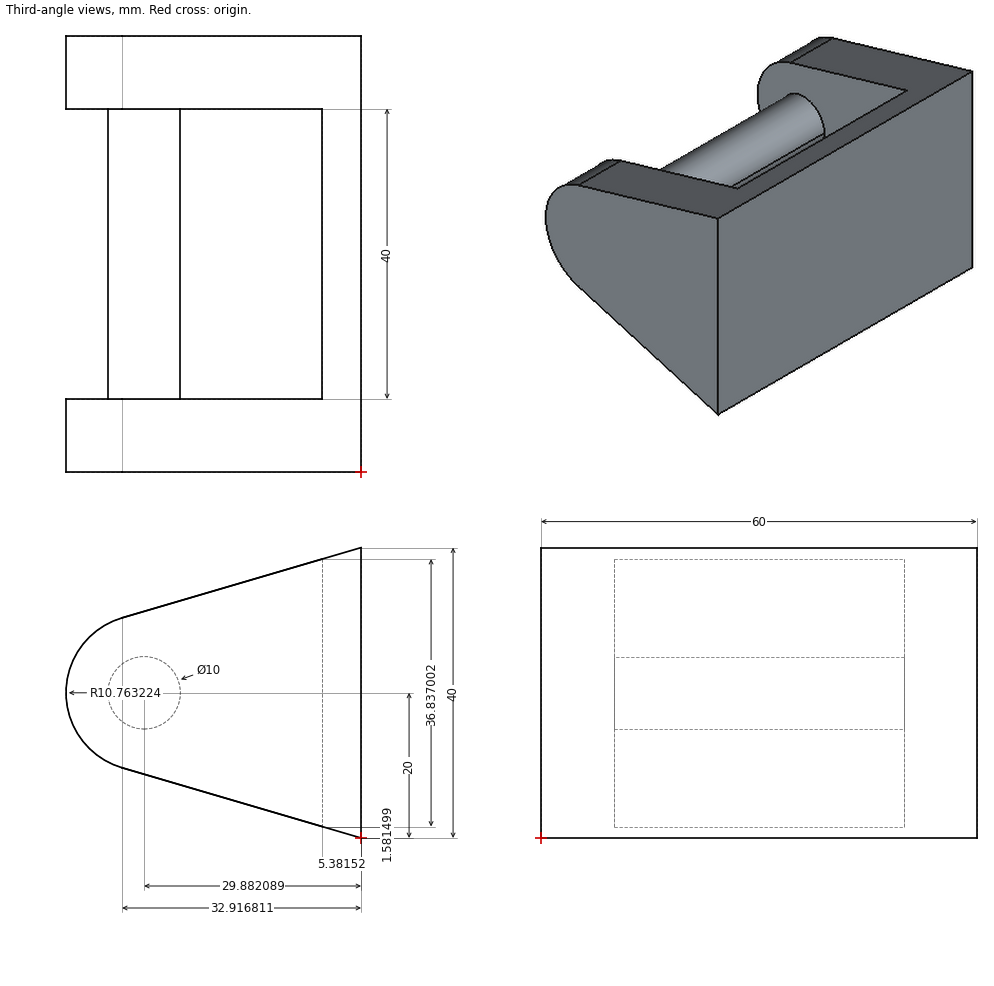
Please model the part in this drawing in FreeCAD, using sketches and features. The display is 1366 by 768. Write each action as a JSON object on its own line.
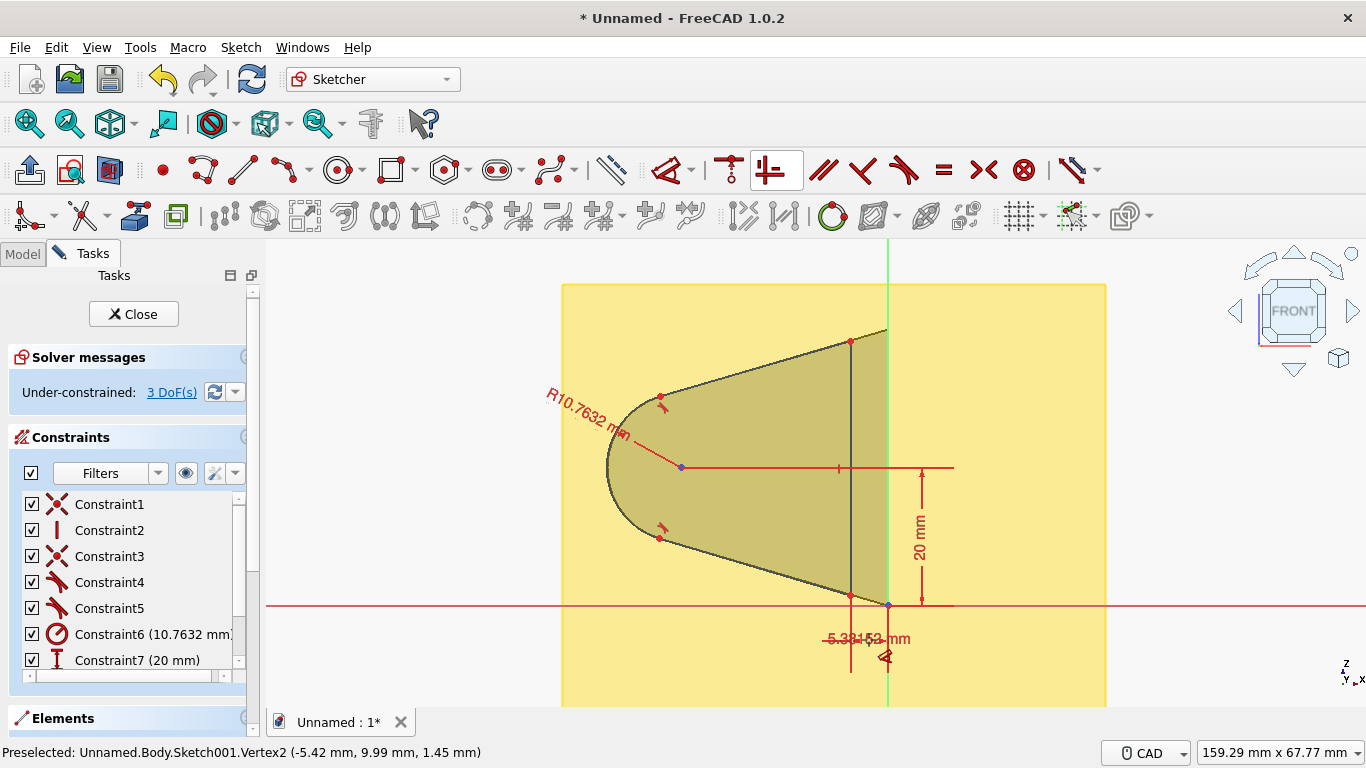
{"action": "left_click", "coordinate": [851, 519]}
{"action": "left_click", "coordinate": [817, 468]}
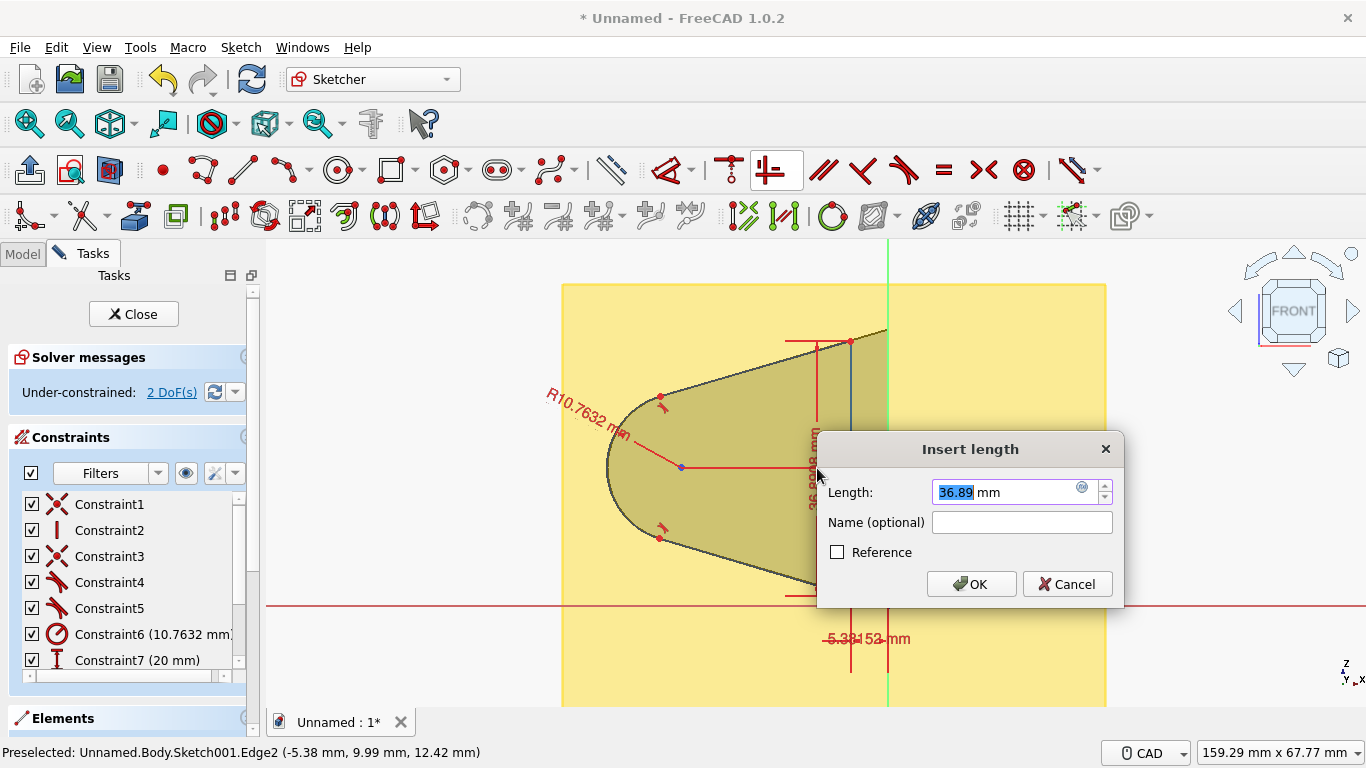
{"action": "type", "text": "36.837002"}
{"action": "key", "text": "Return"}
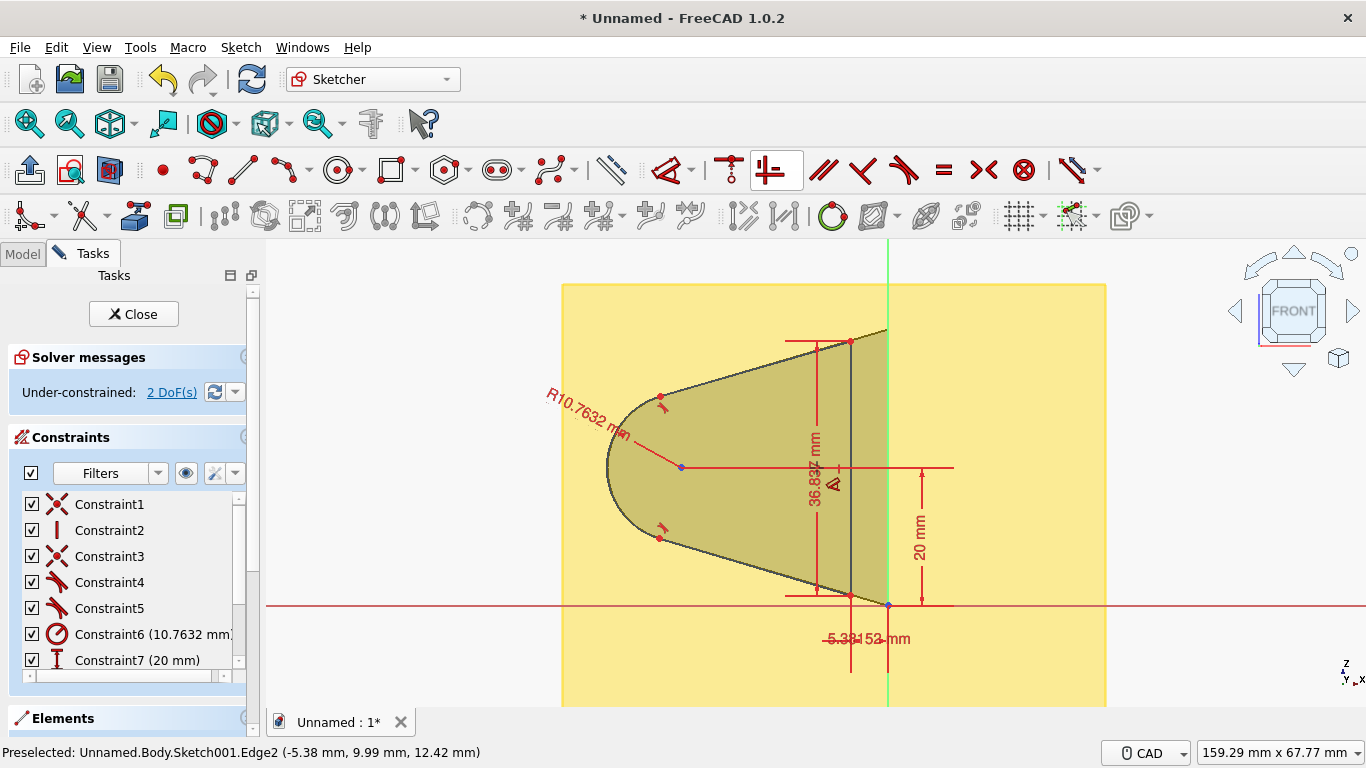
{"action": "scroll", "coordinate": [851, 596], "scroll_direction": "up", "scroll_amount": 7}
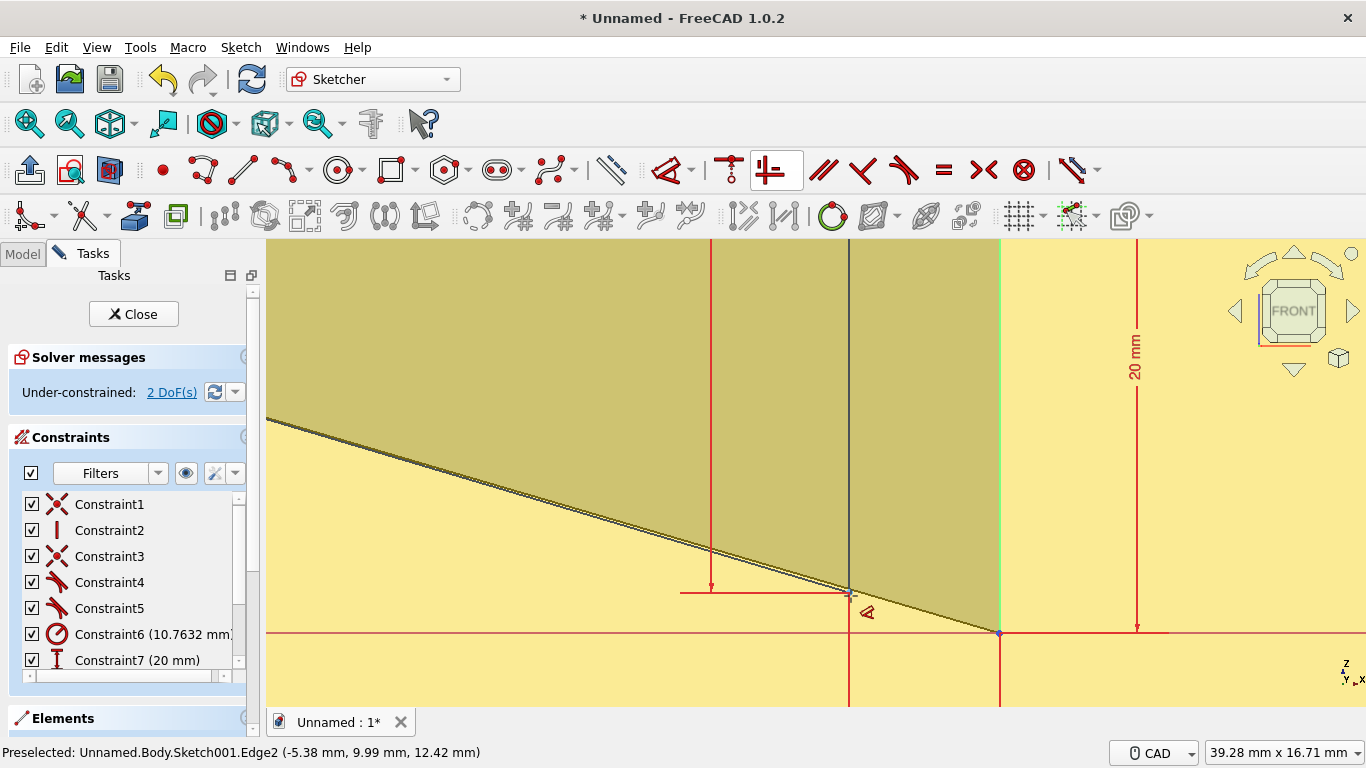
{"action": "left_click", "coordinate": [849, 593]}
{"action": "left_click", "coordinate": [1034, 613]}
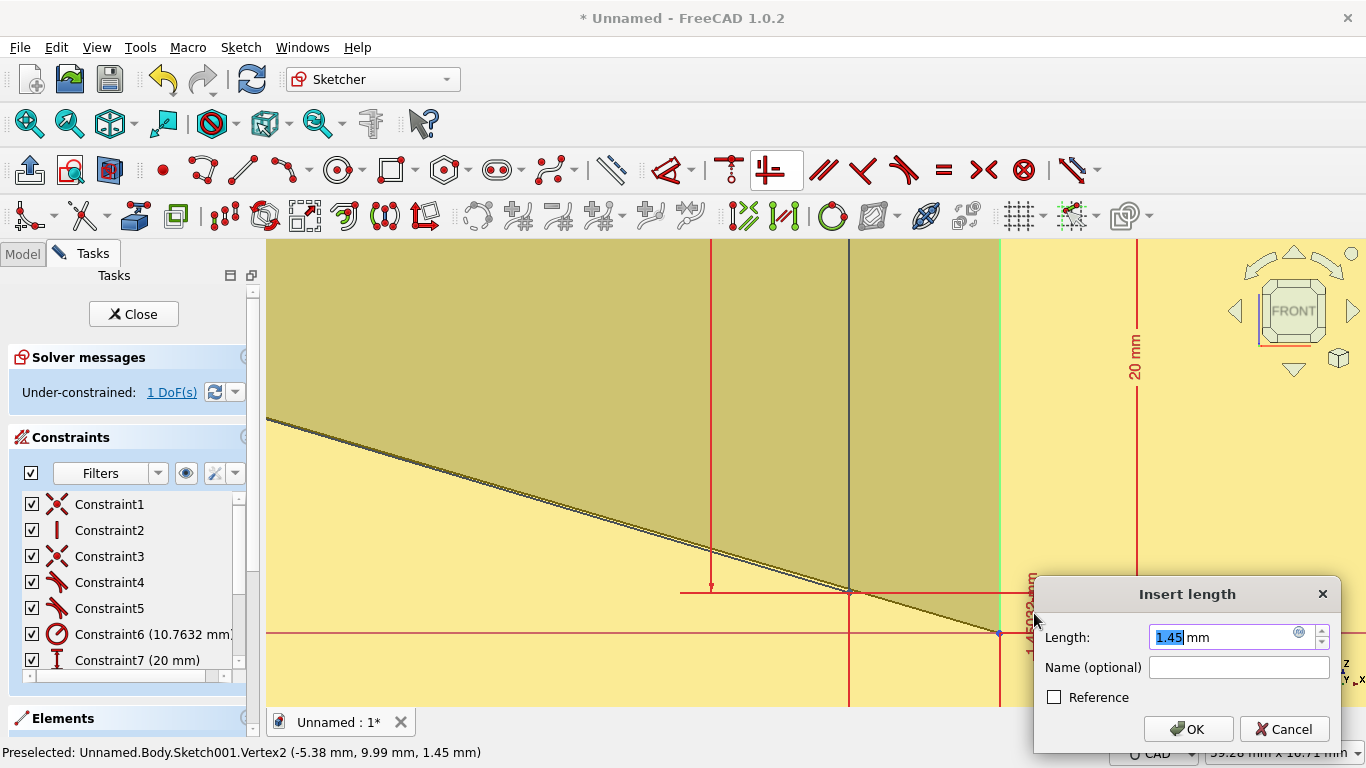
{"action": "type", "text": "1.581499"}
{"action": "key", "text": "Return"}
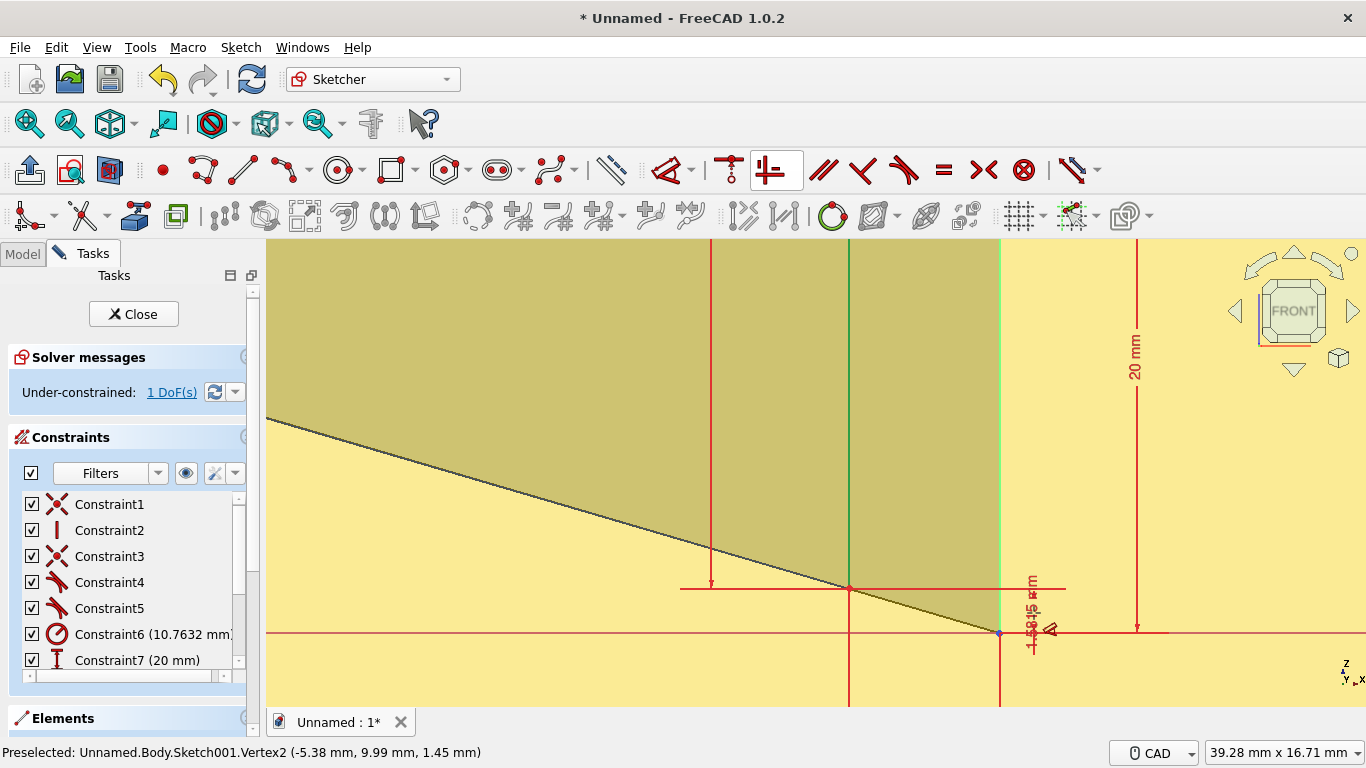
{"action": "scroll", "coordinate": [851, 597], "scroll_direction": "down", "scroll_amount": 7}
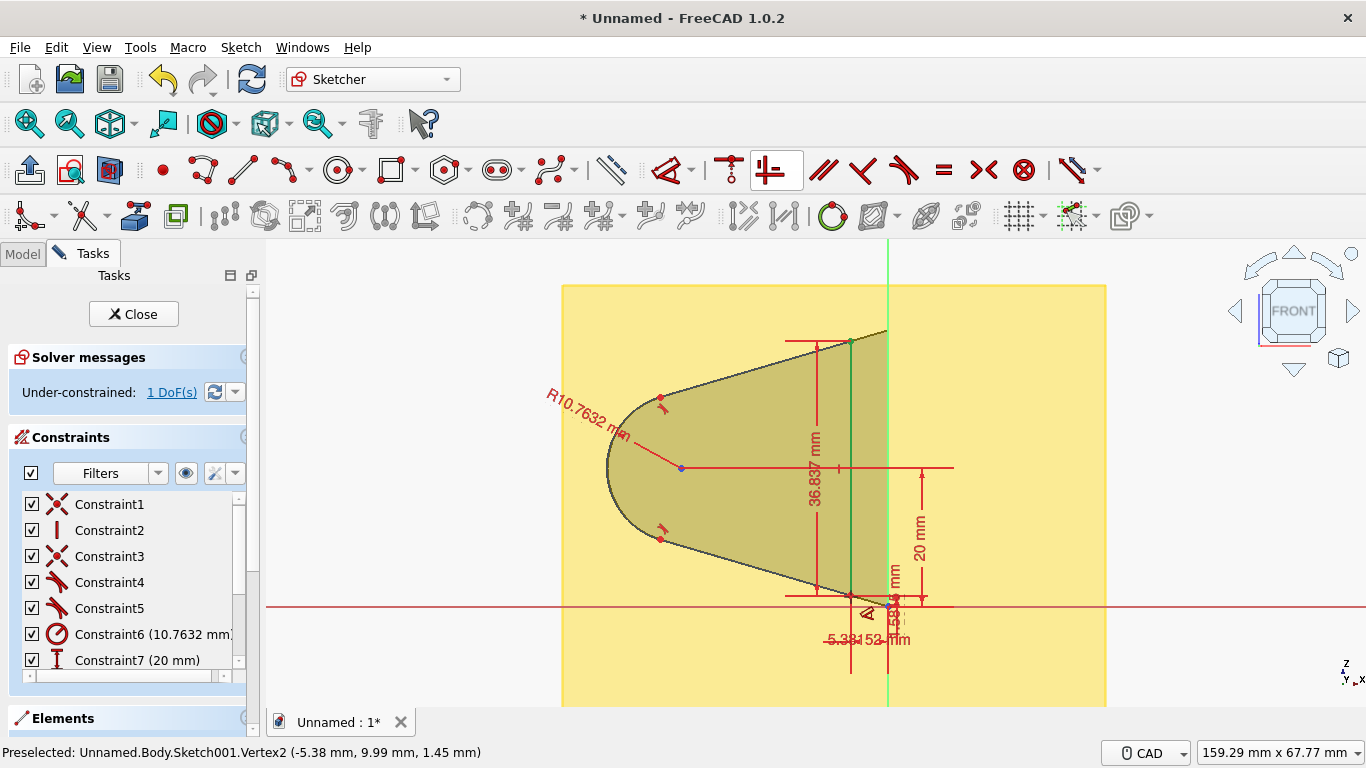
{"action": "left_click", "coordinate": [660, 540]}
{"action": "left_click", "coordinate": [774, 641]}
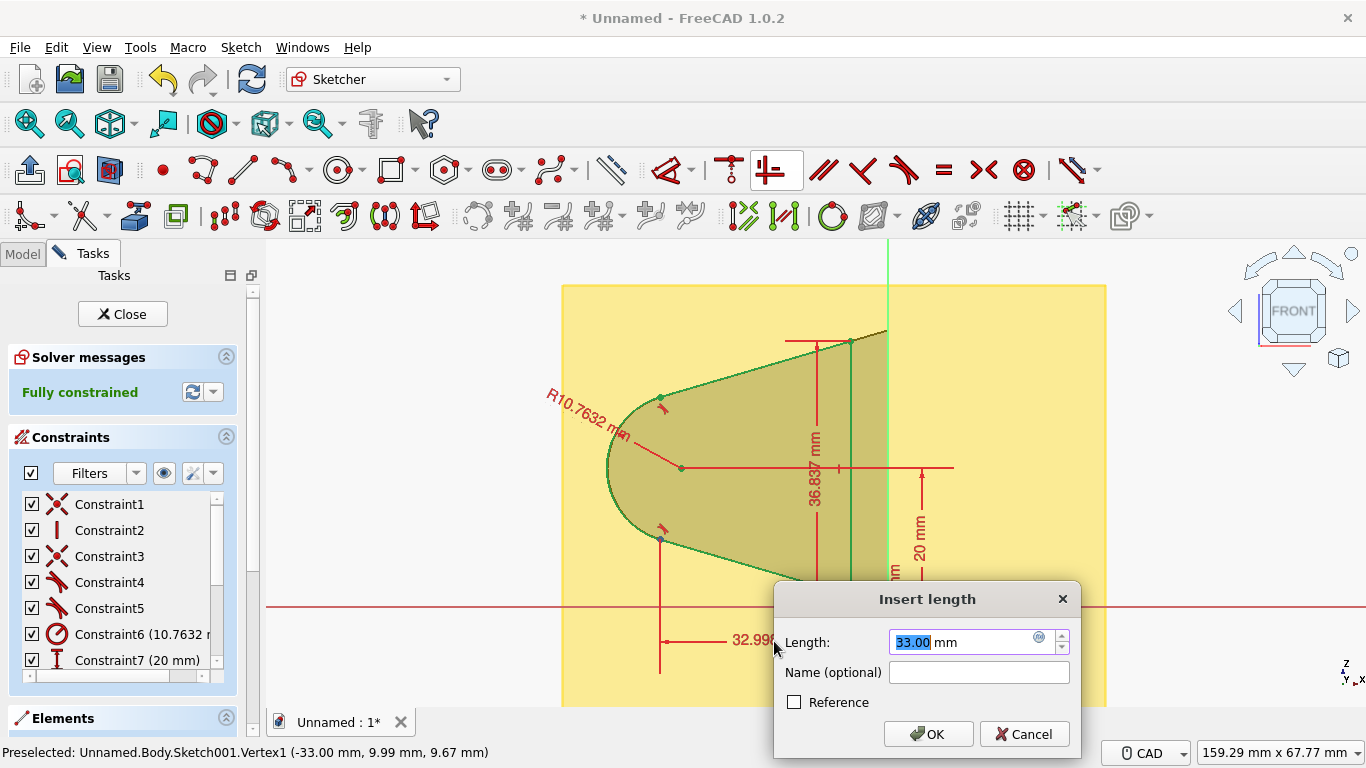
{"action": "type", "text": "32.916811"}
{"action": "key", "text": "Return"}
{"action": "key", "text": "Escape"}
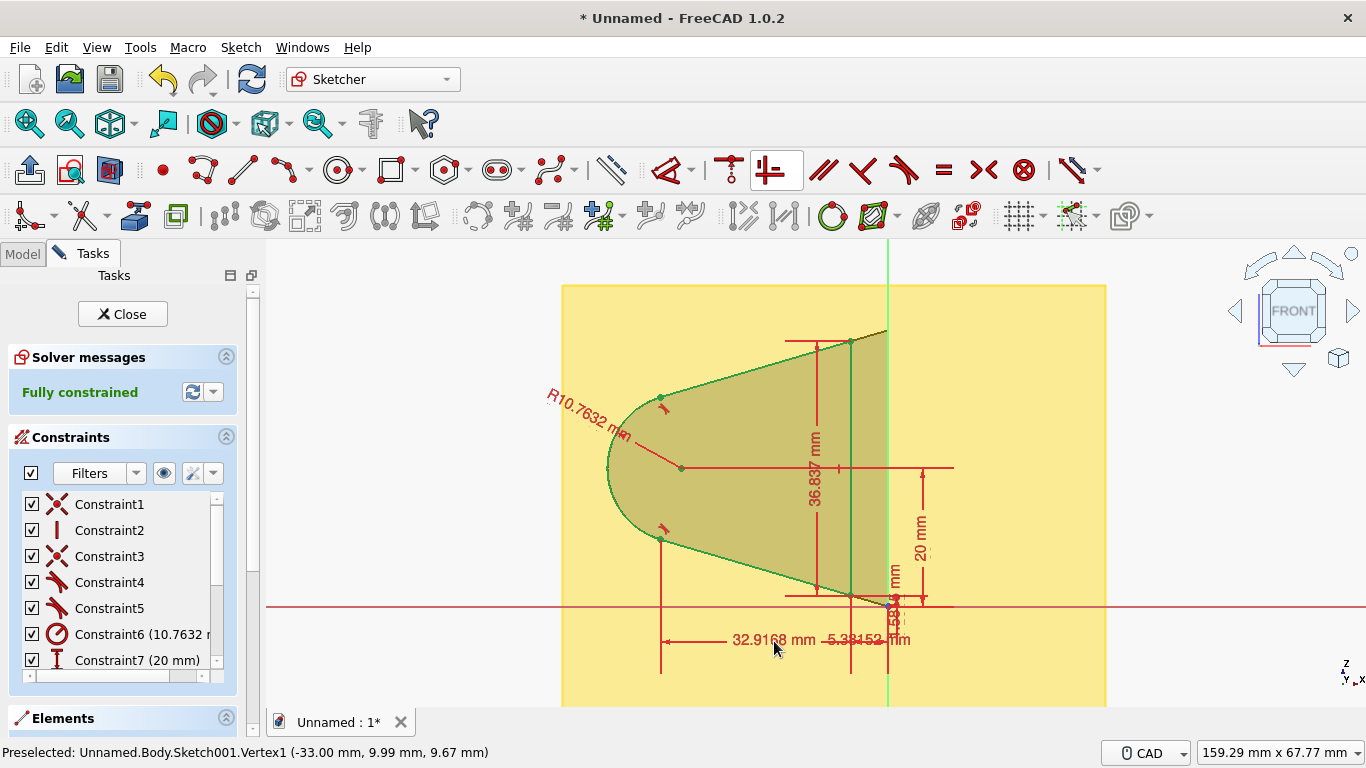
{"action": "left_click", "coordinate": [123, 314]}